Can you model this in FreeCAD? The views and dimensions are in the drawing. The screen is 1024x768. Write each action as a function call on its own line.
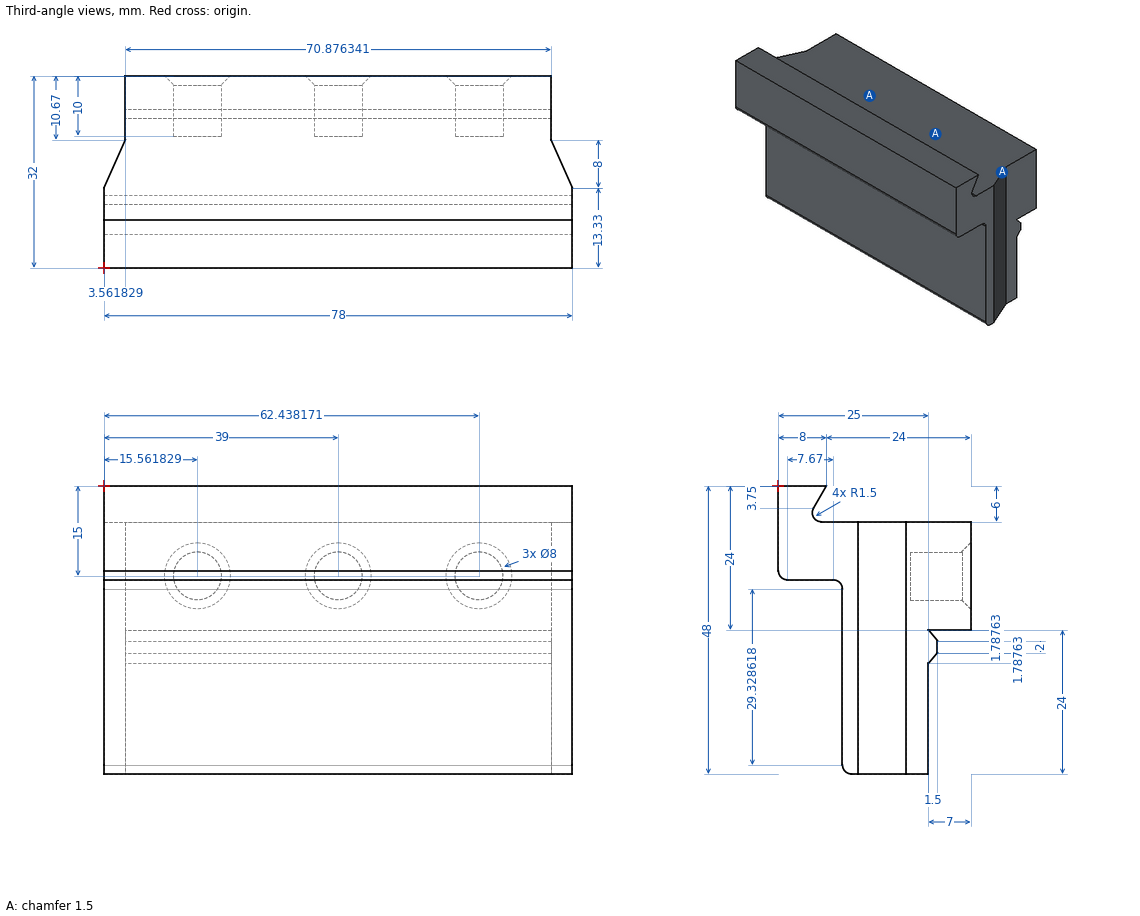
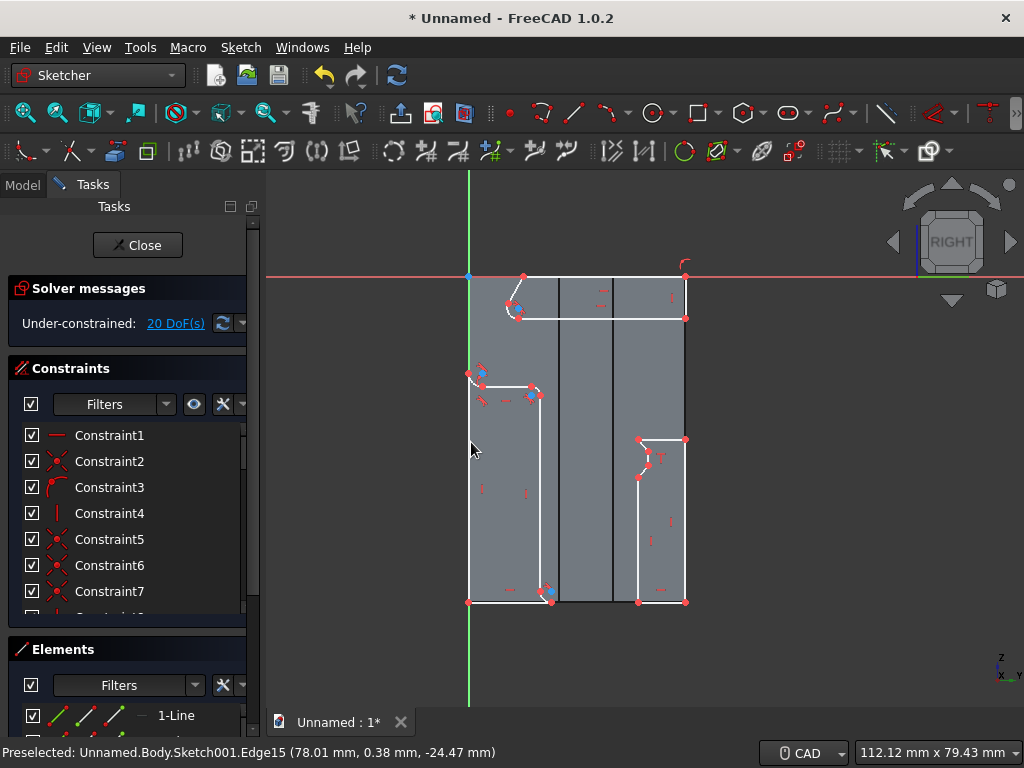
scroll(507, 310, up, 4)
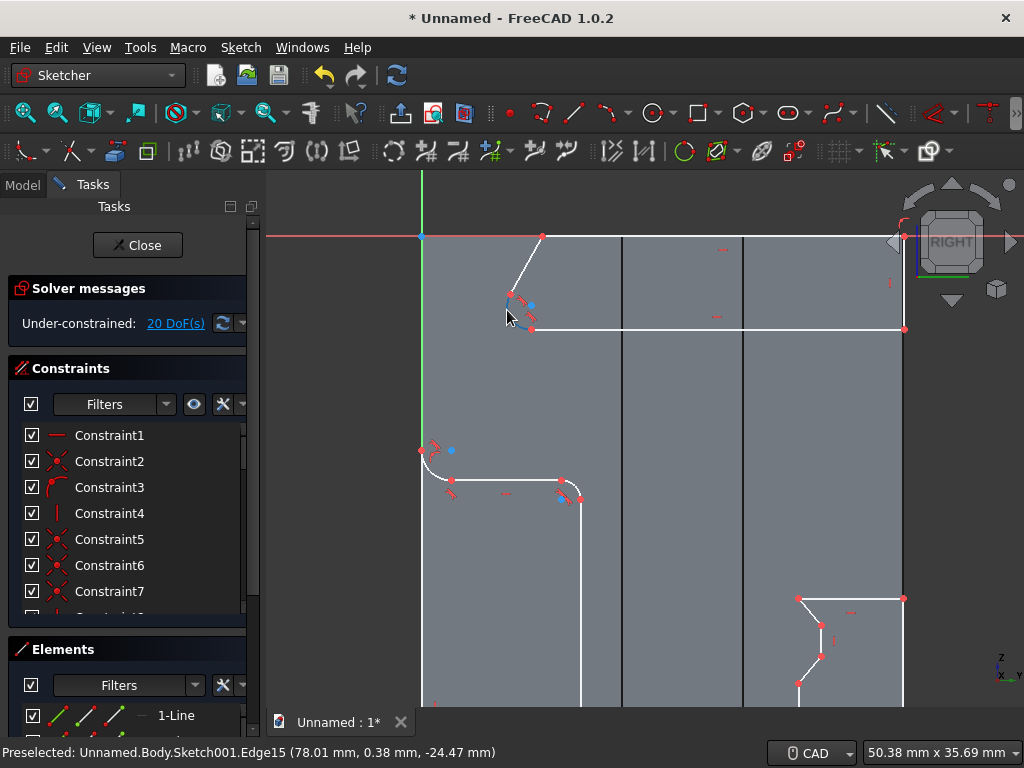
click(508, 309)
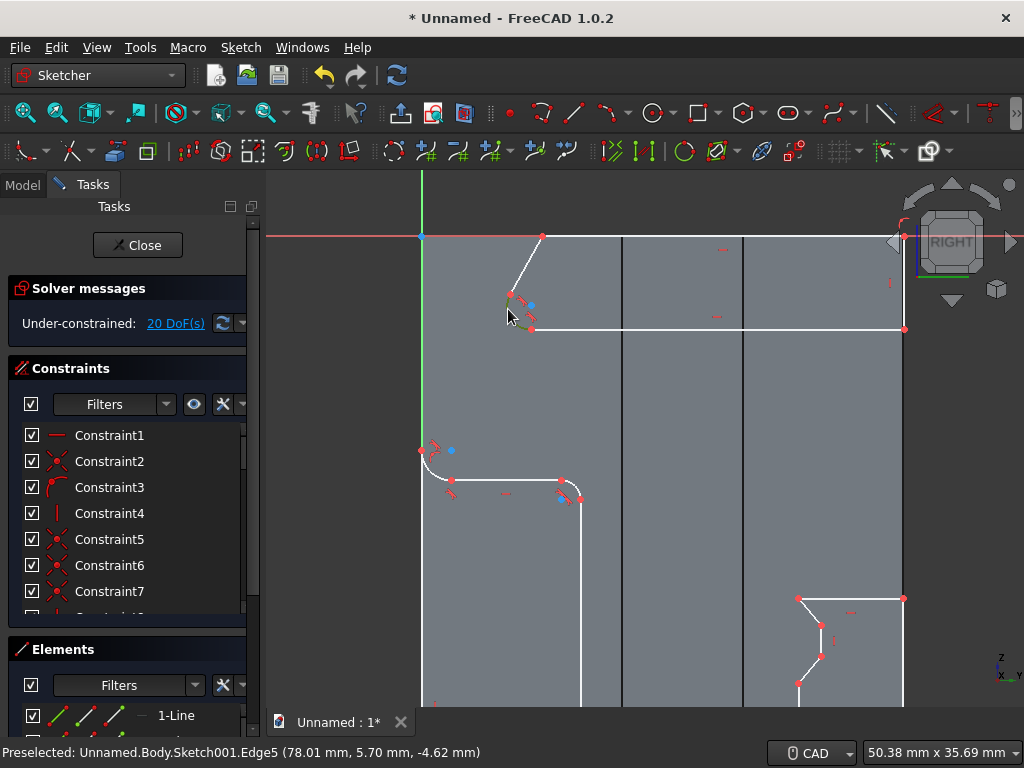
scroll(579, 491, up, 3)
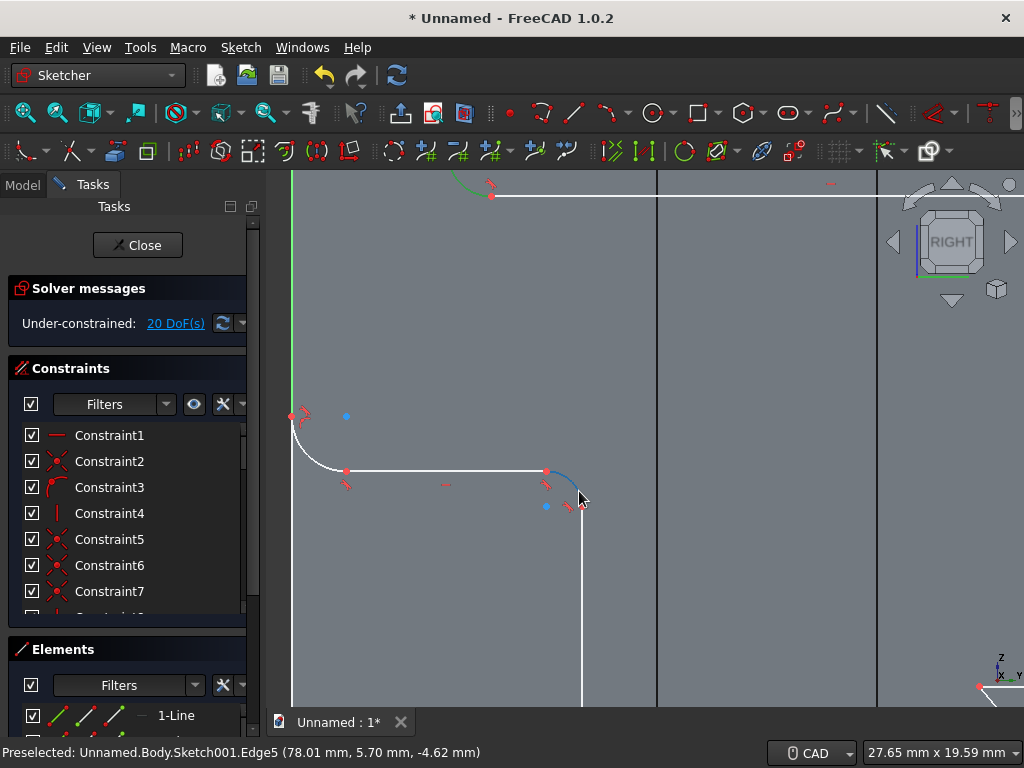
click(578, 491)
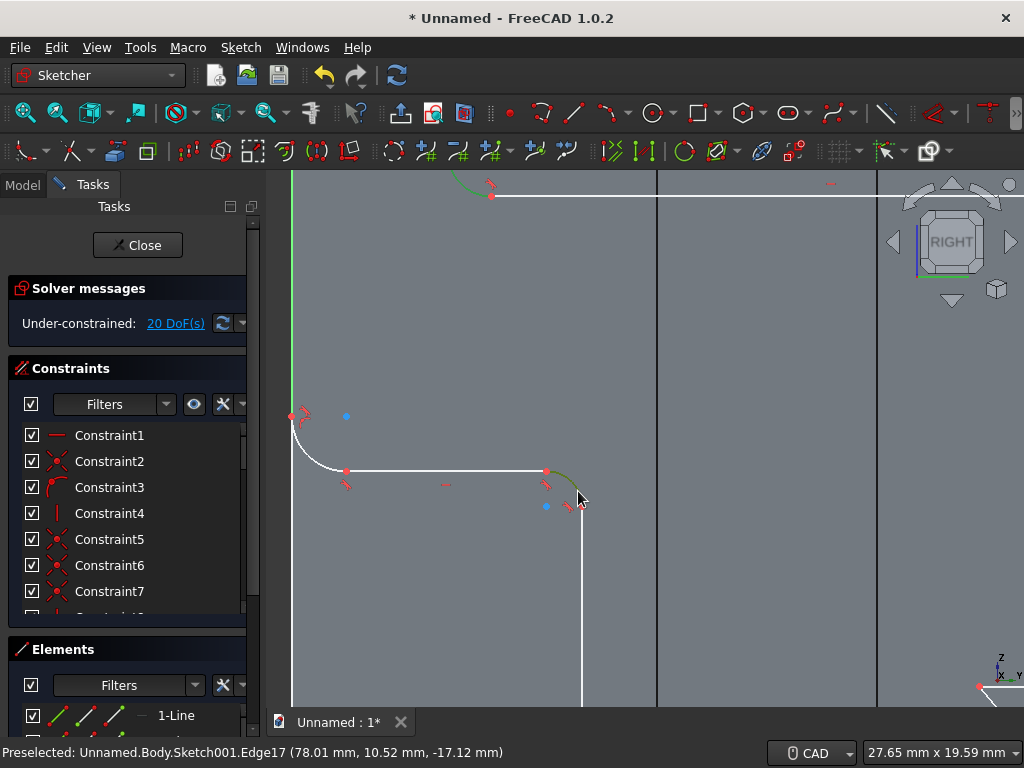
click(322, 465)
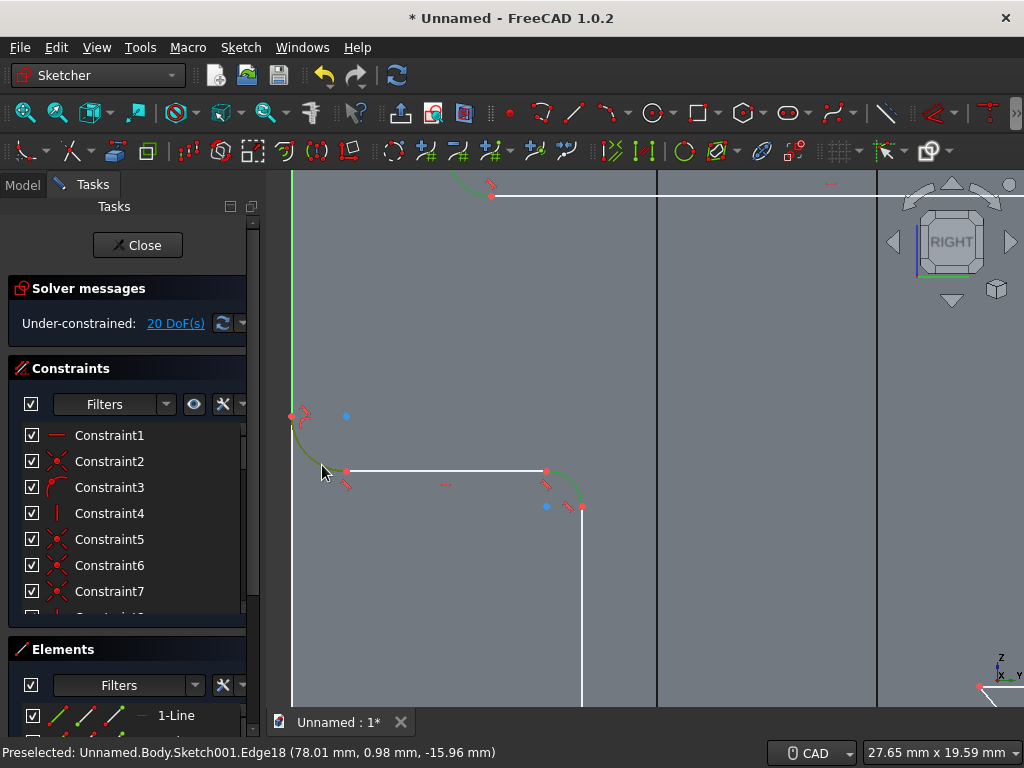
scroll(526, 358, down, 7)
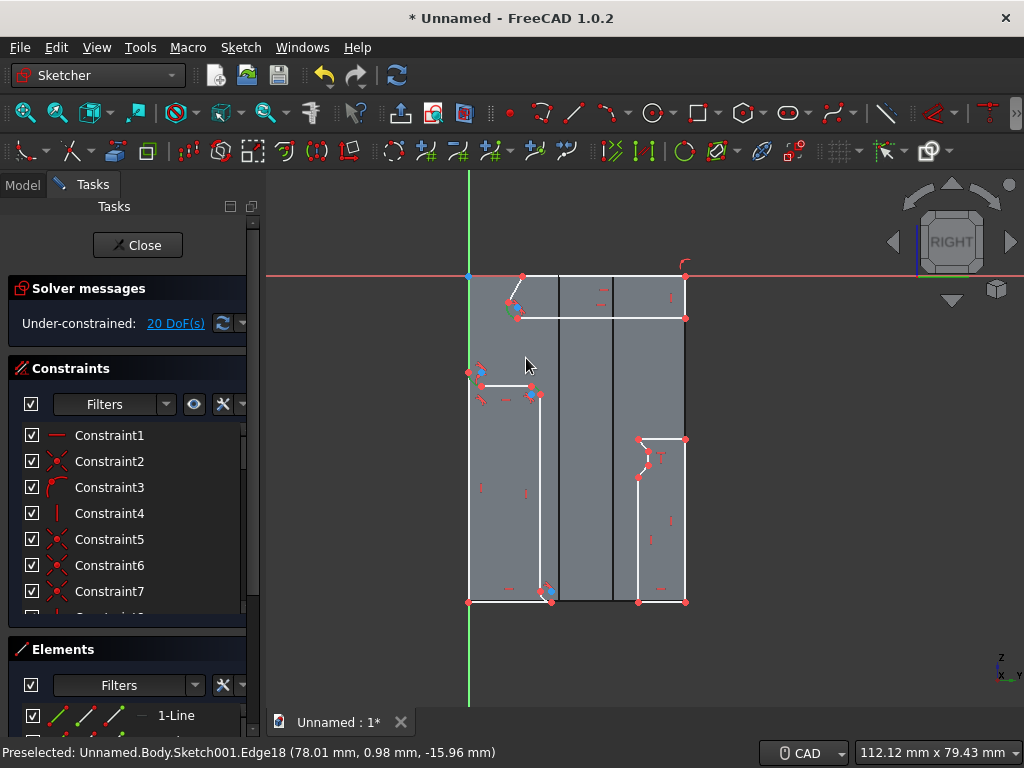
scroll(541, 596, up, 5)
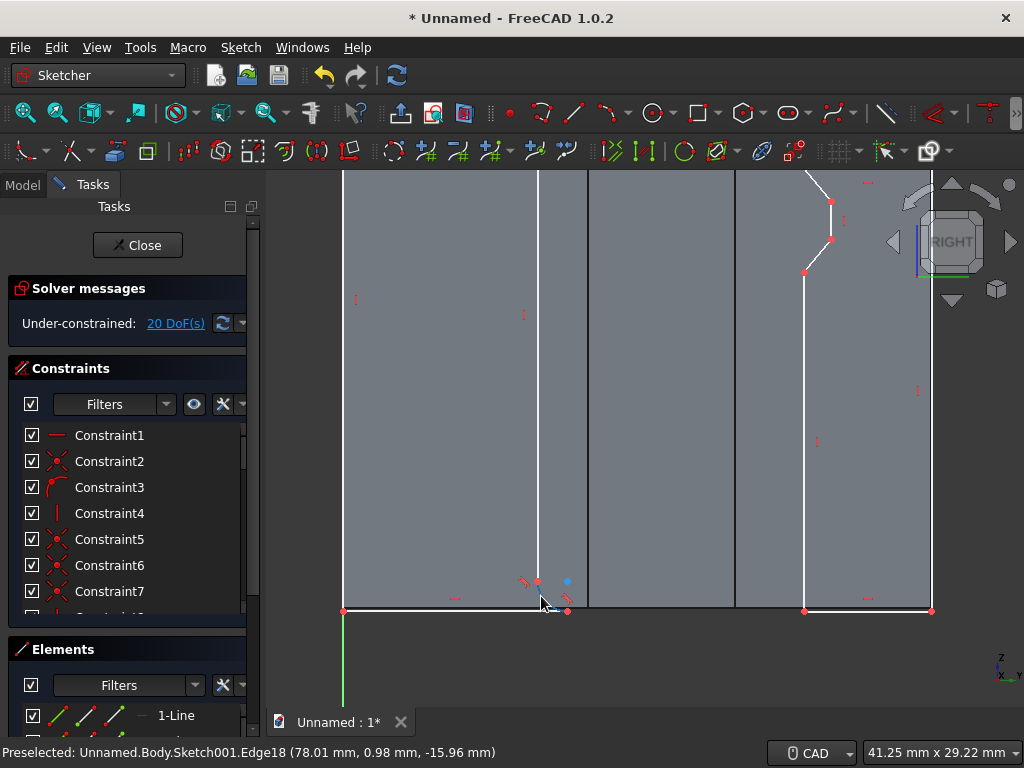
click(541, 595)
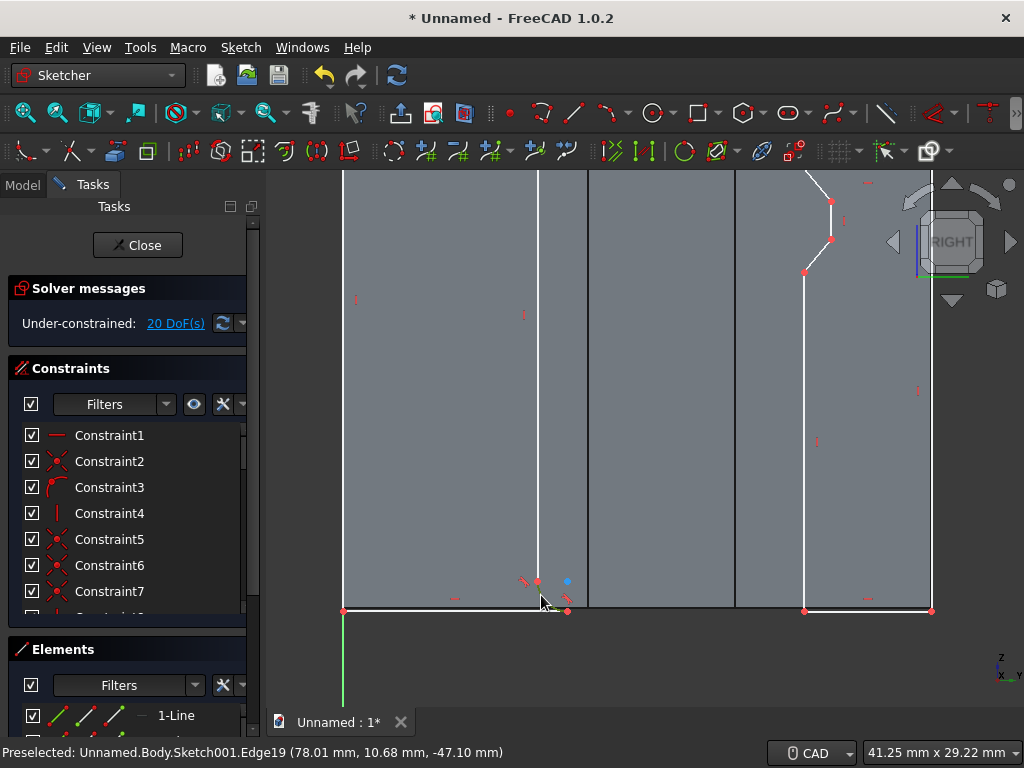
key(e)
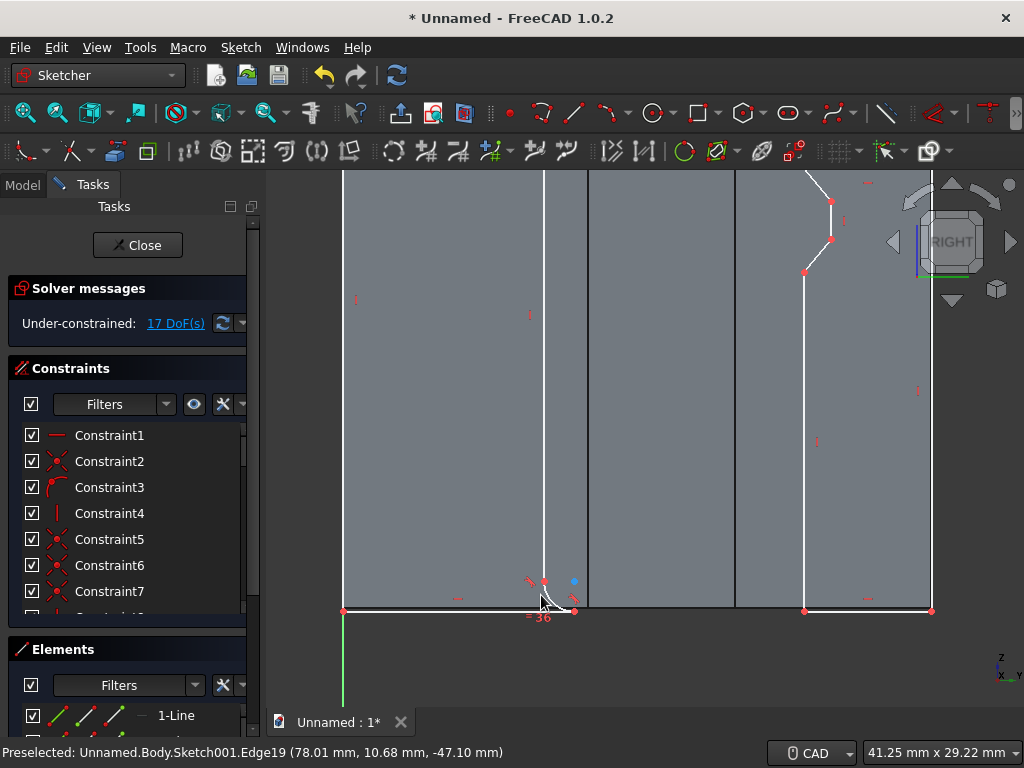
click(934, 114)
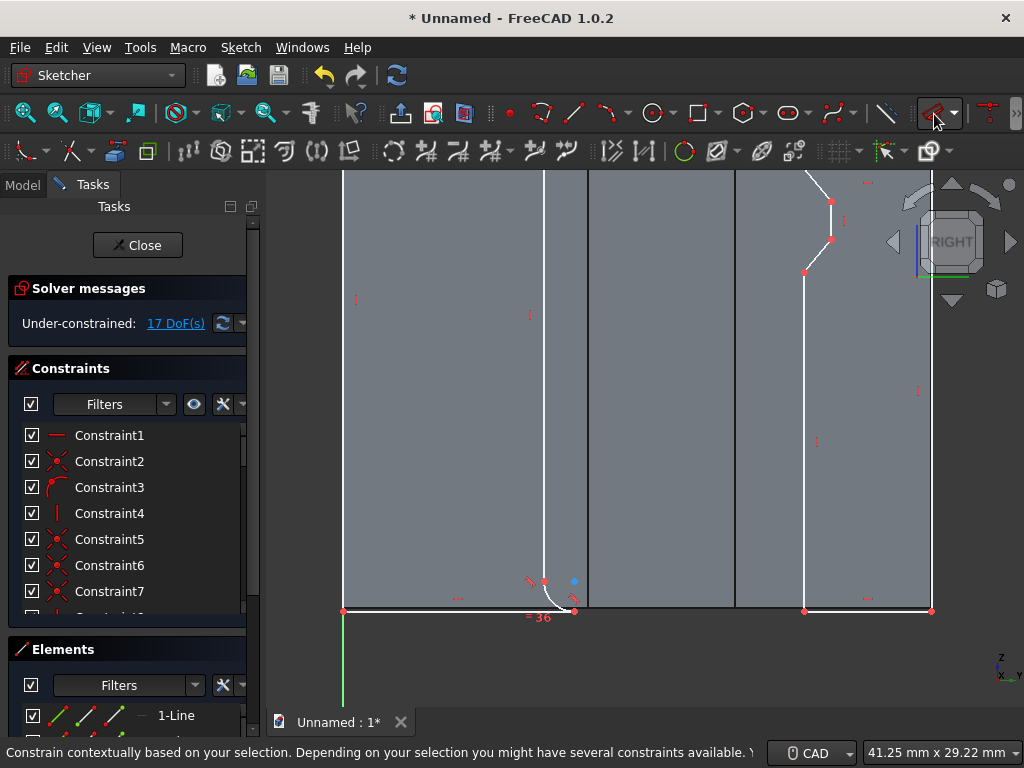
scroll(541, 596, down, 5)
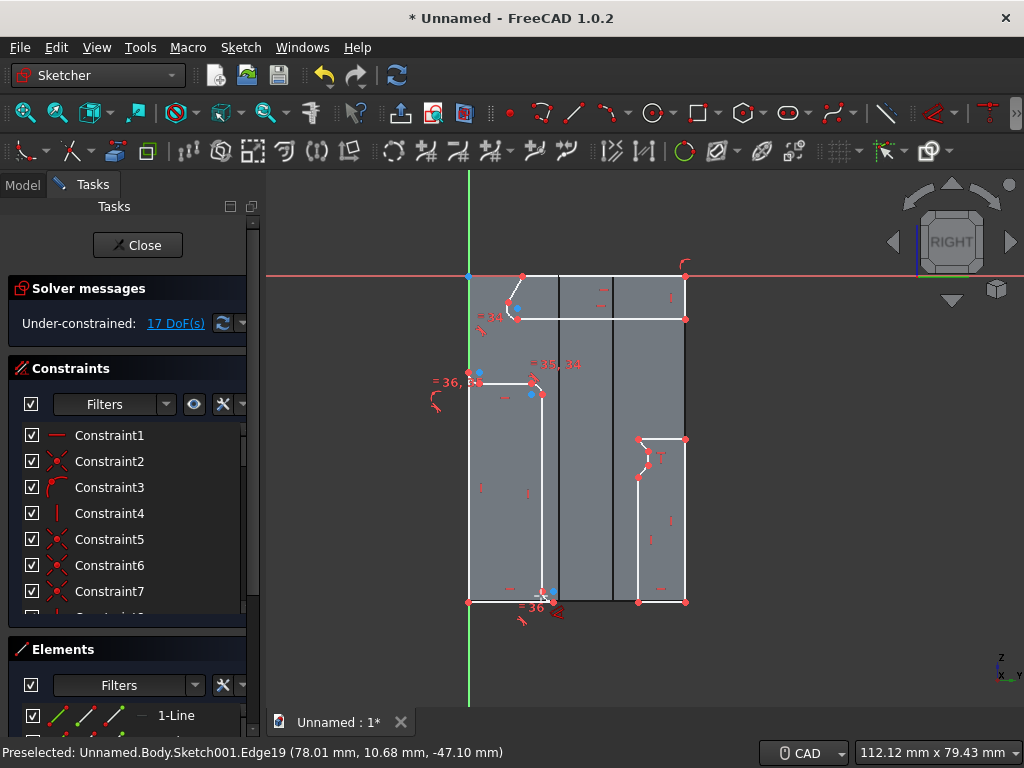
scroll(507, 310, up, 7)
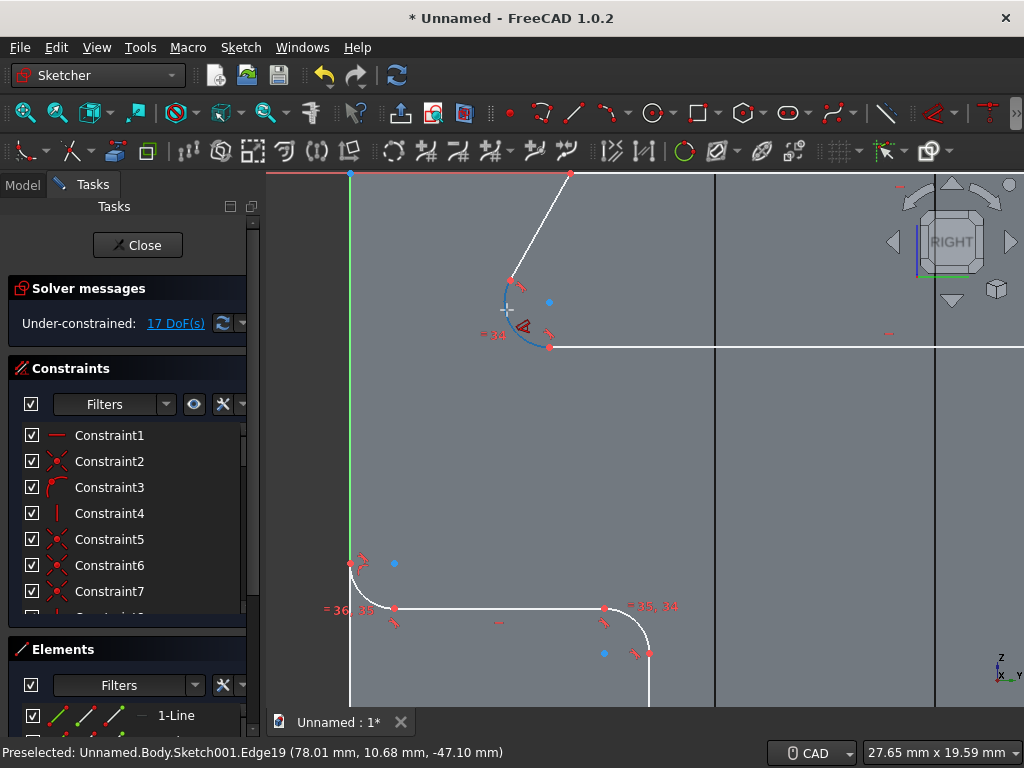
click(505, 307)
click(473, 310)